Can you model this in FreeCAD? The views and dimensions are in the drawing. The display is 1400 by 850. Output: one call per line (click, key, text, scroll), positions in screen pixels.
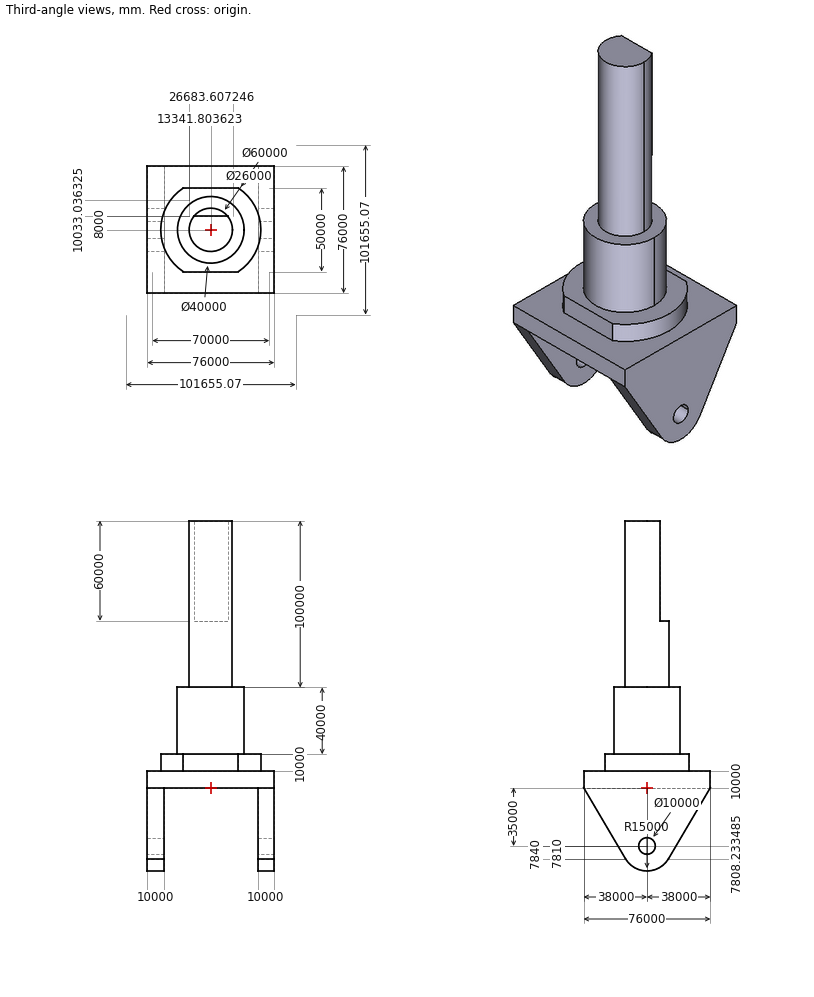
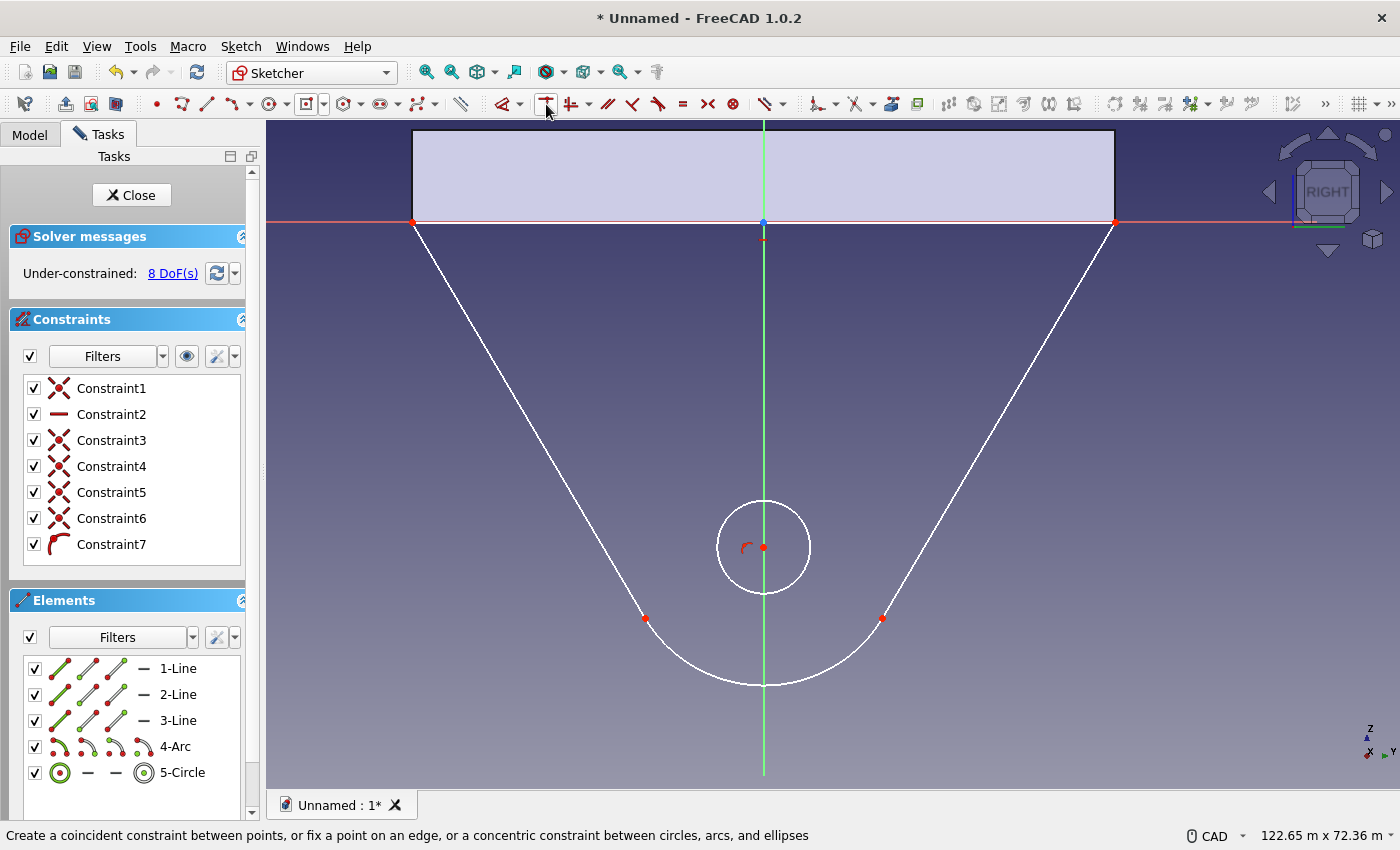
click(502, 104)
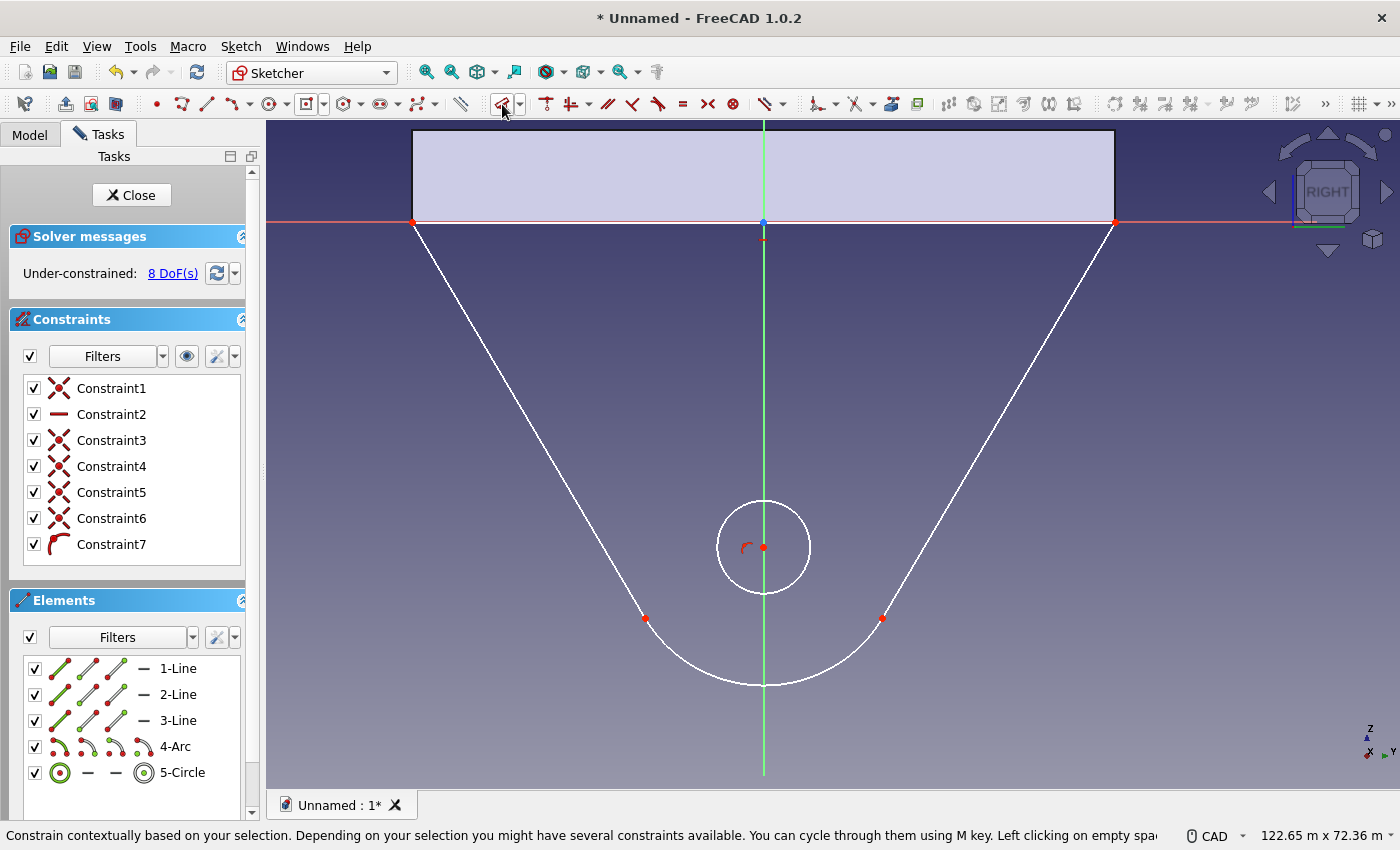
click(709, 674)
click(696, 703)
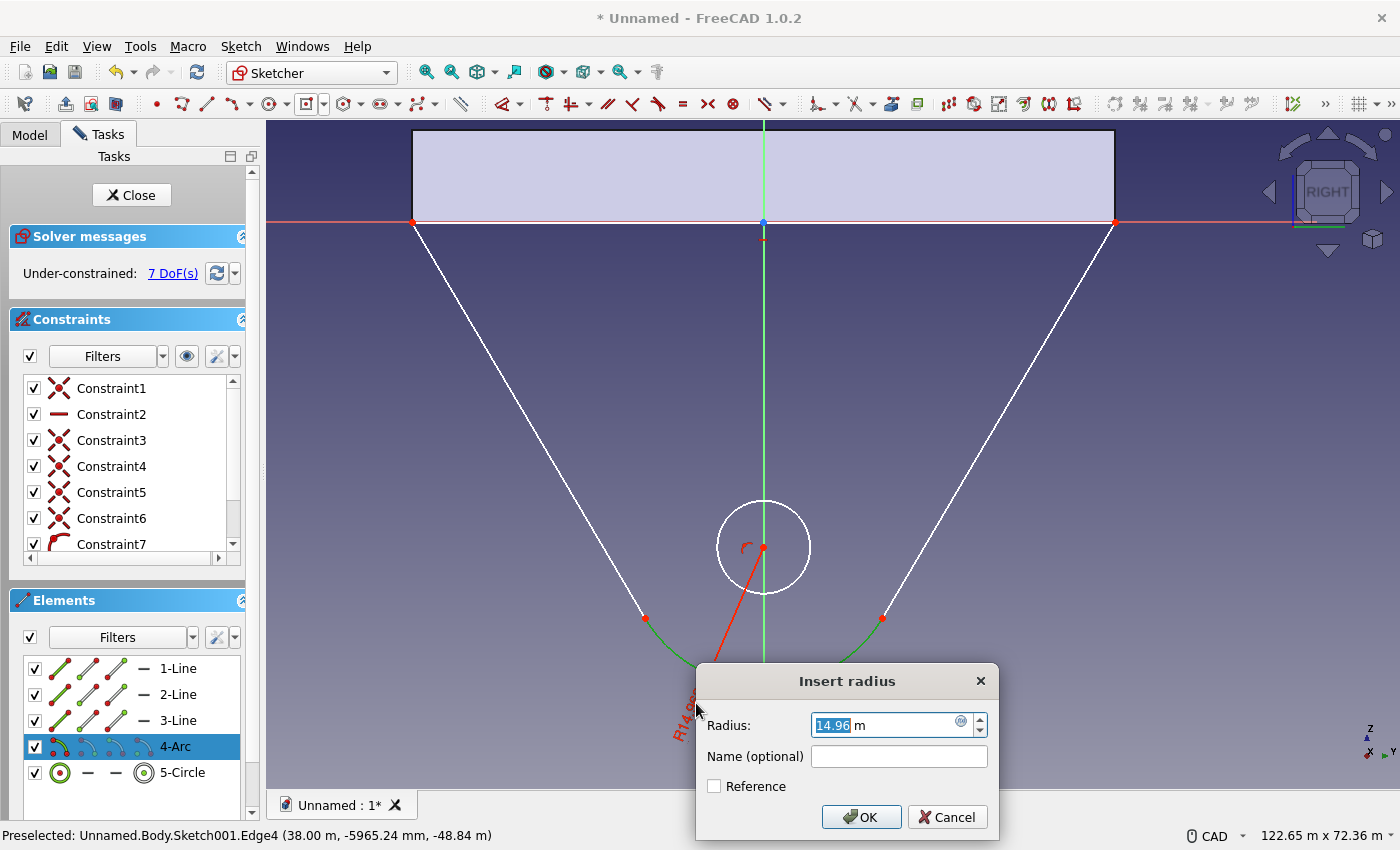
key(ctrl+a)
text(15000 mm)
key(Return)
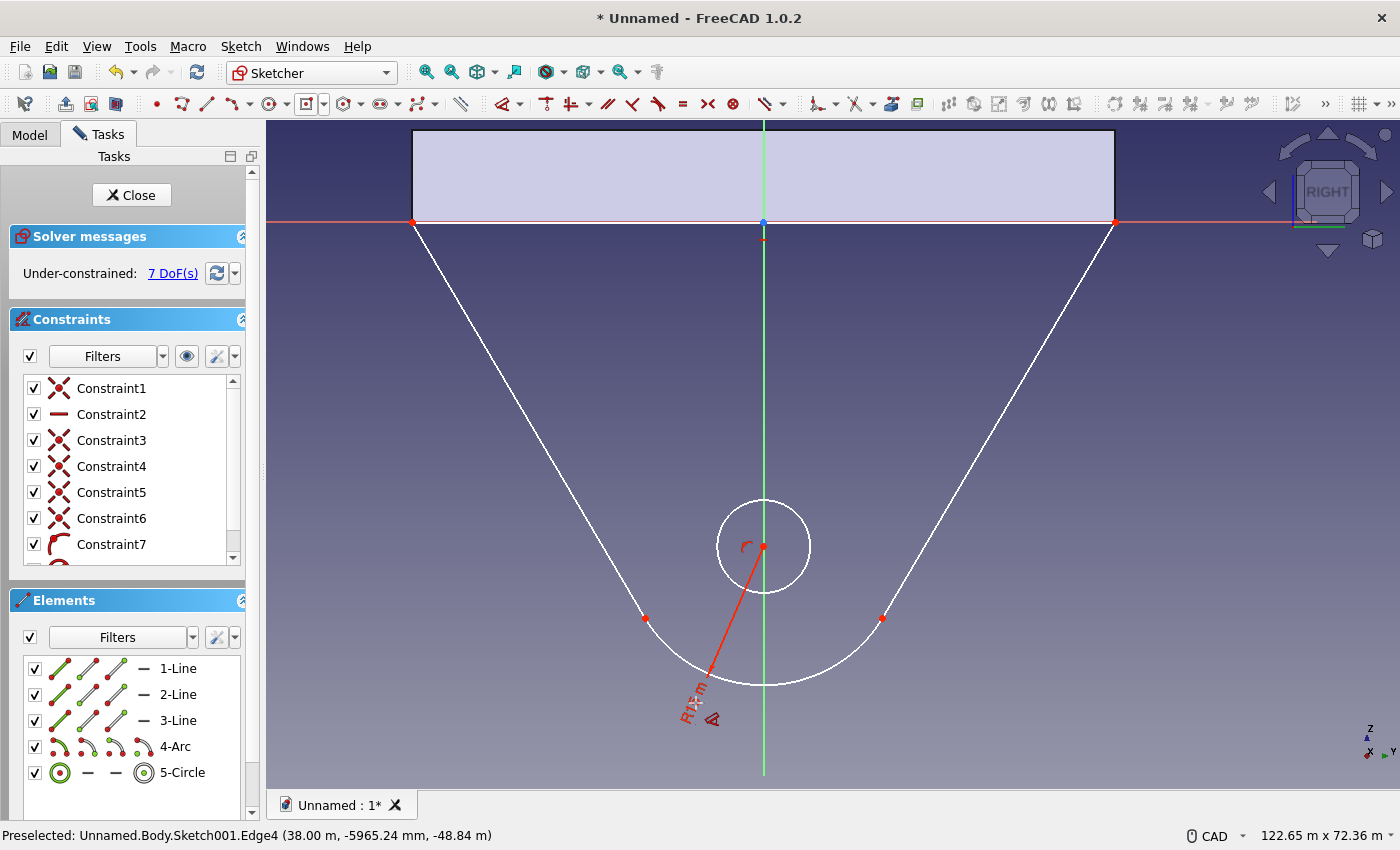
click(796, 514)
click(819, 491)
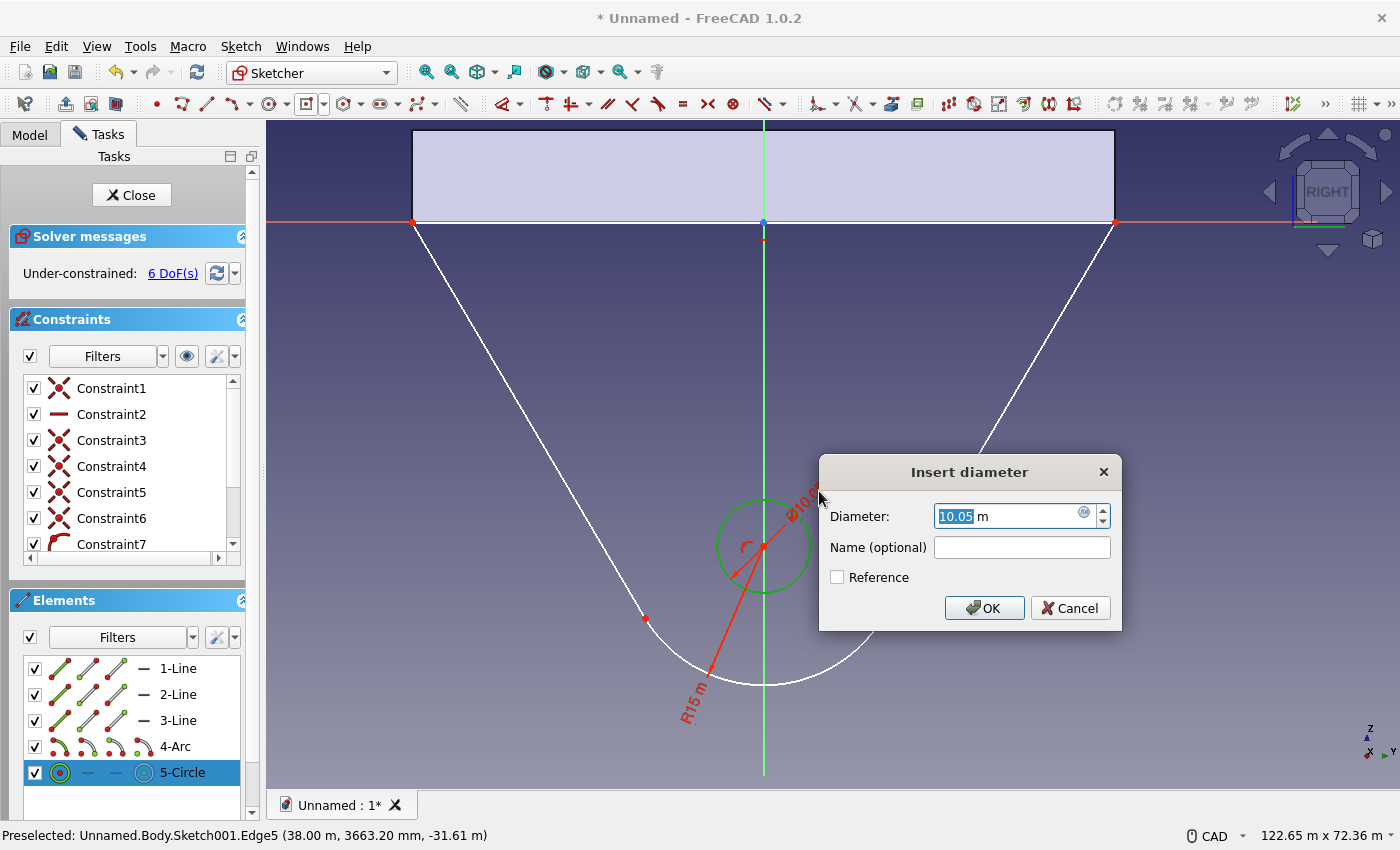
key(ctrl+a)
text(10000 mm)
key(Return)
key(Escape)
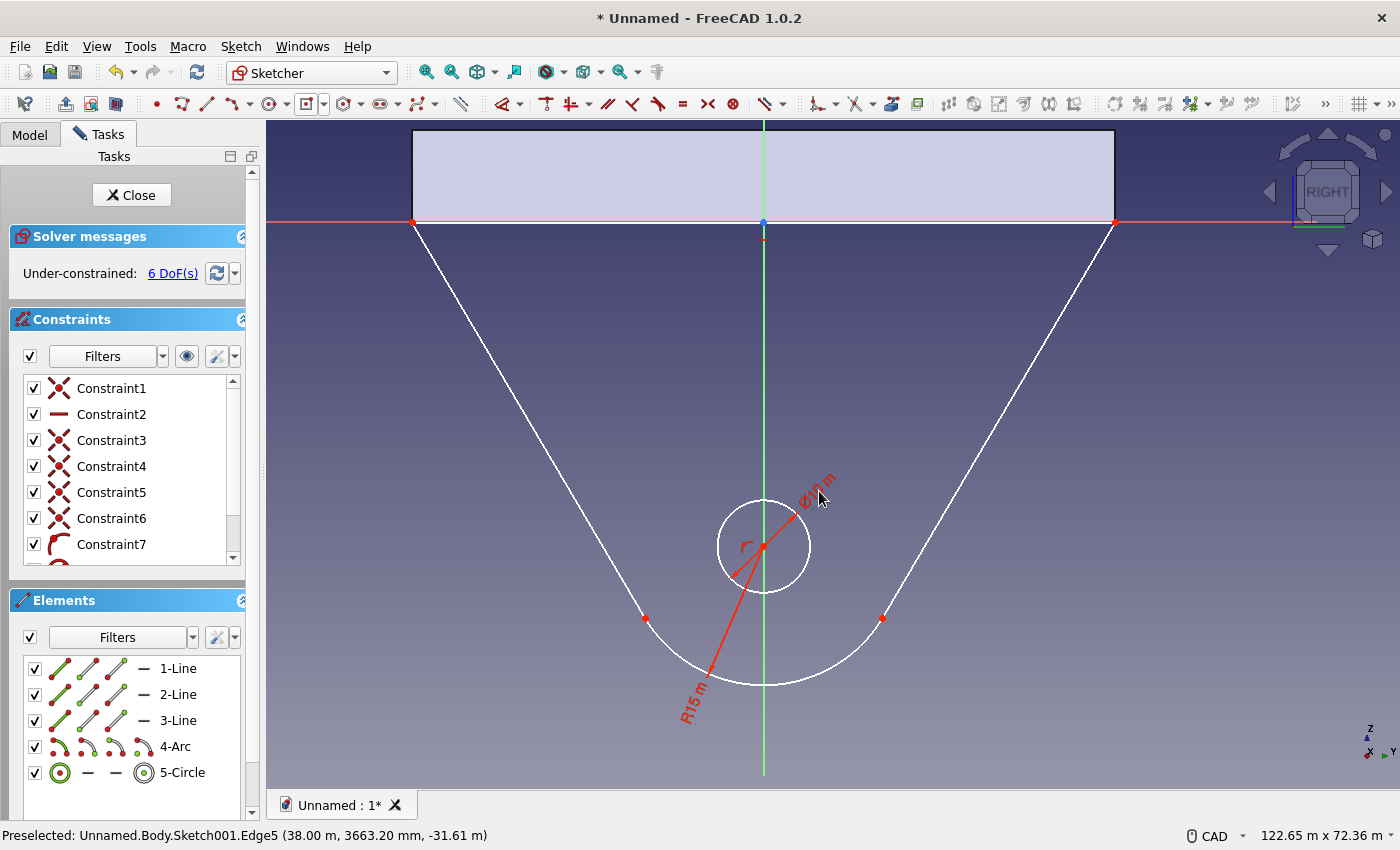
click(1115, 223)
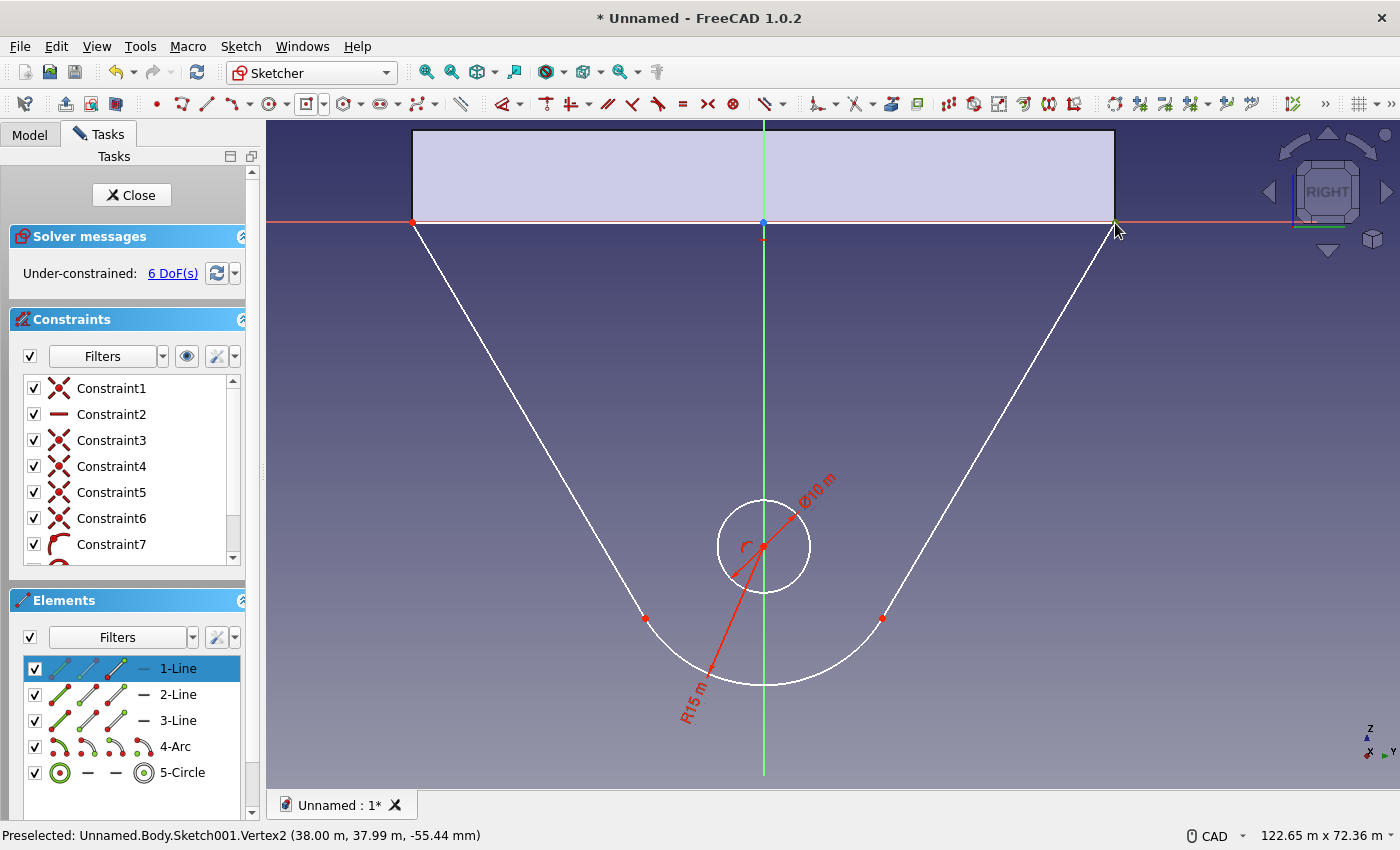
click(361, 222)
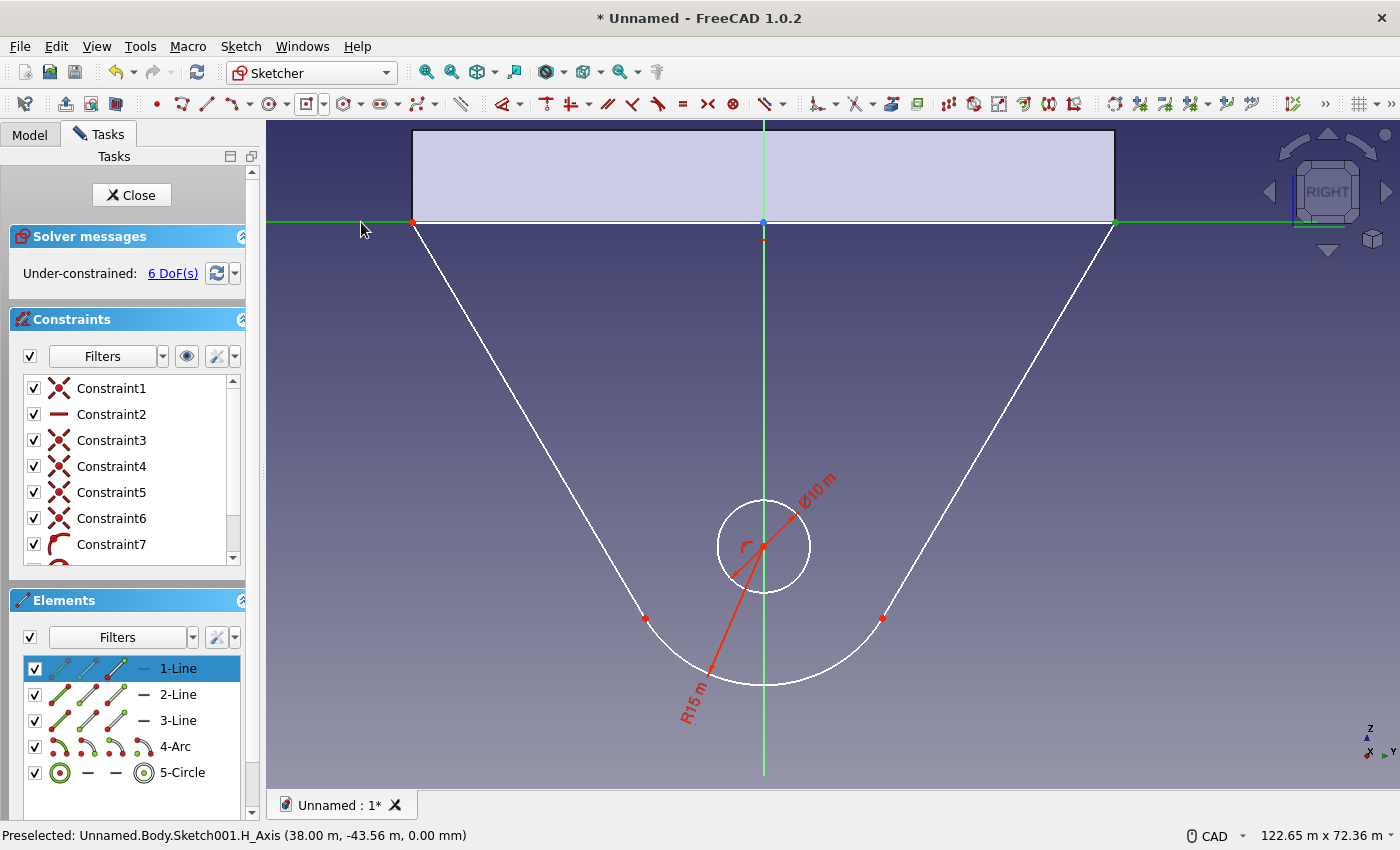
click(546, 104)